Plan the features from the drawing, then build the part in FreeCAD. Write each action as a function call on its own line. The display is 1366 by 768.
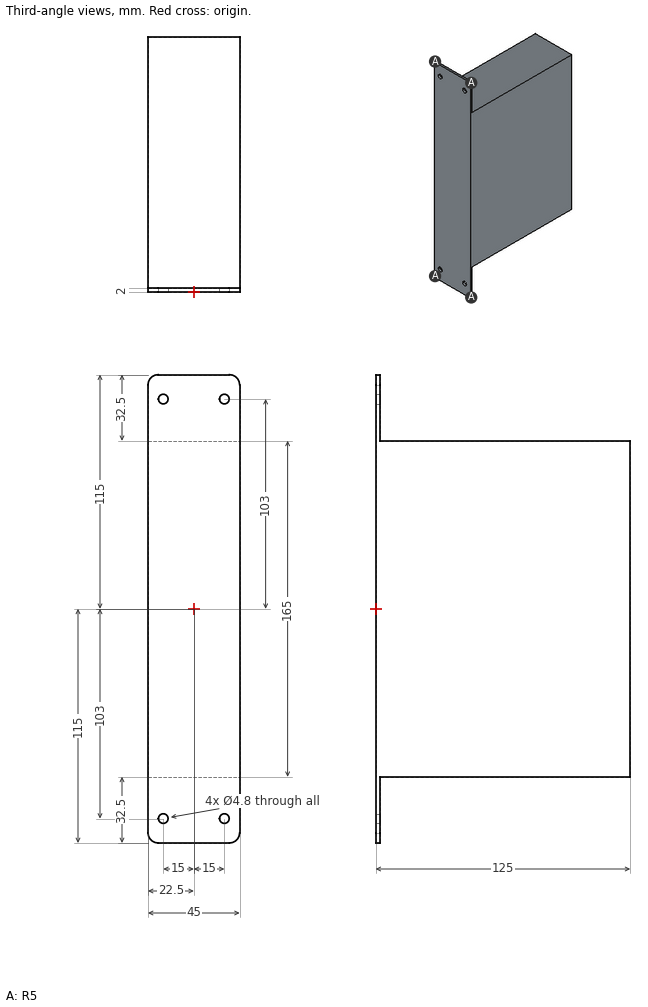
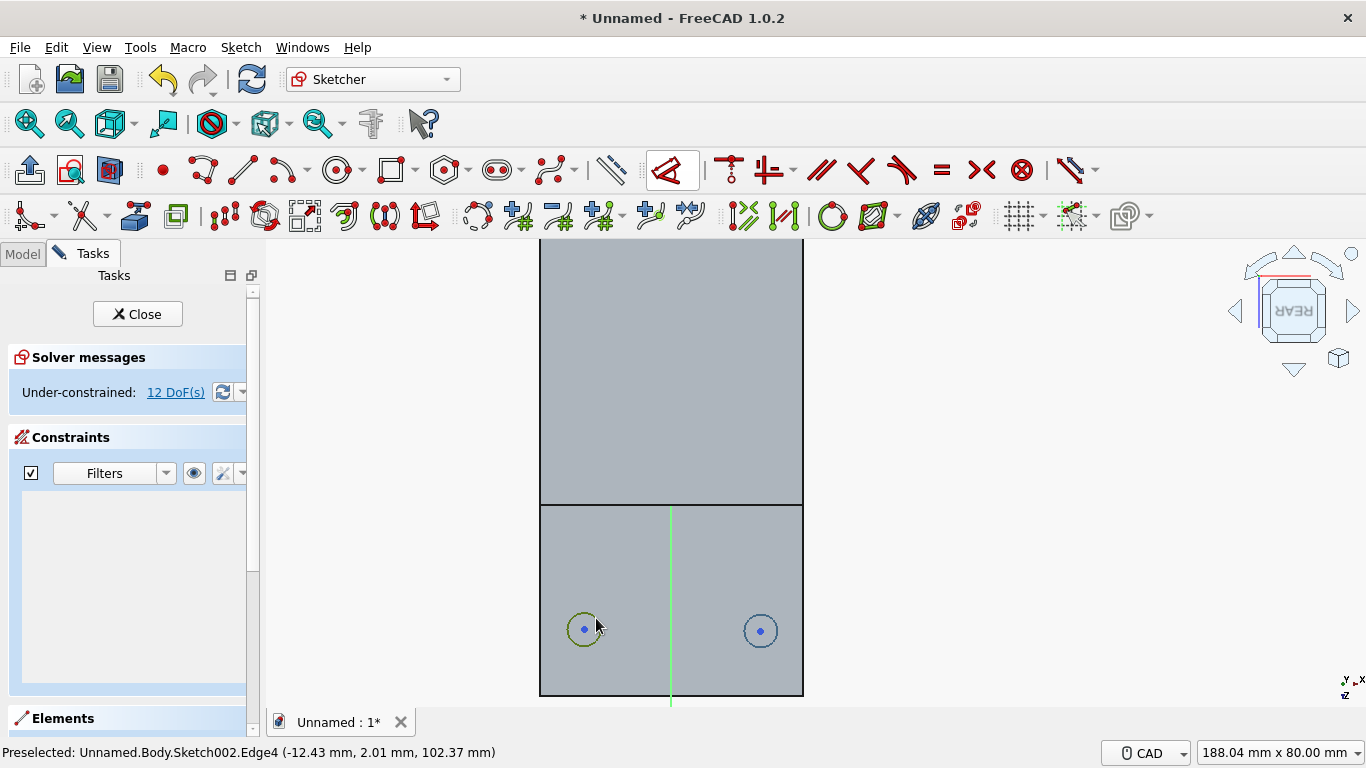
click(942, 170)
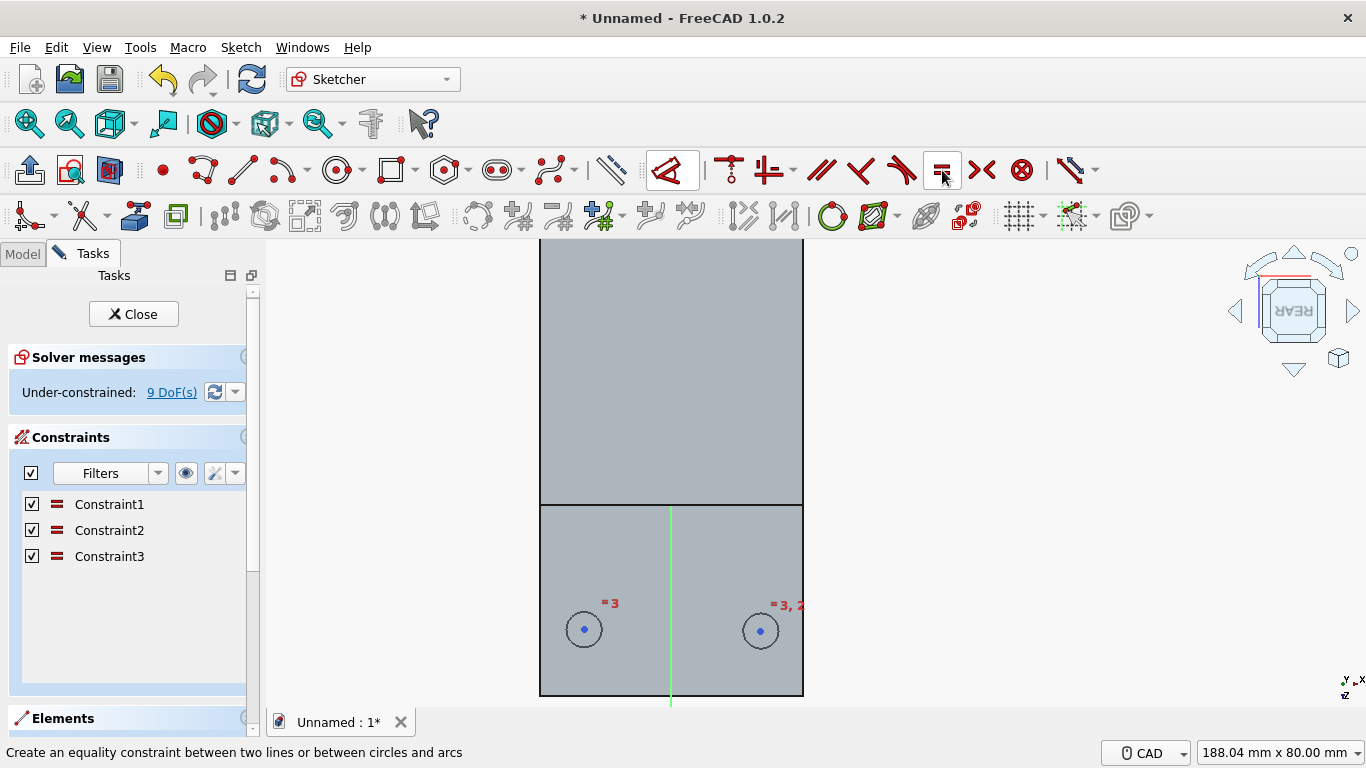
scroll(772, 620, down, 7)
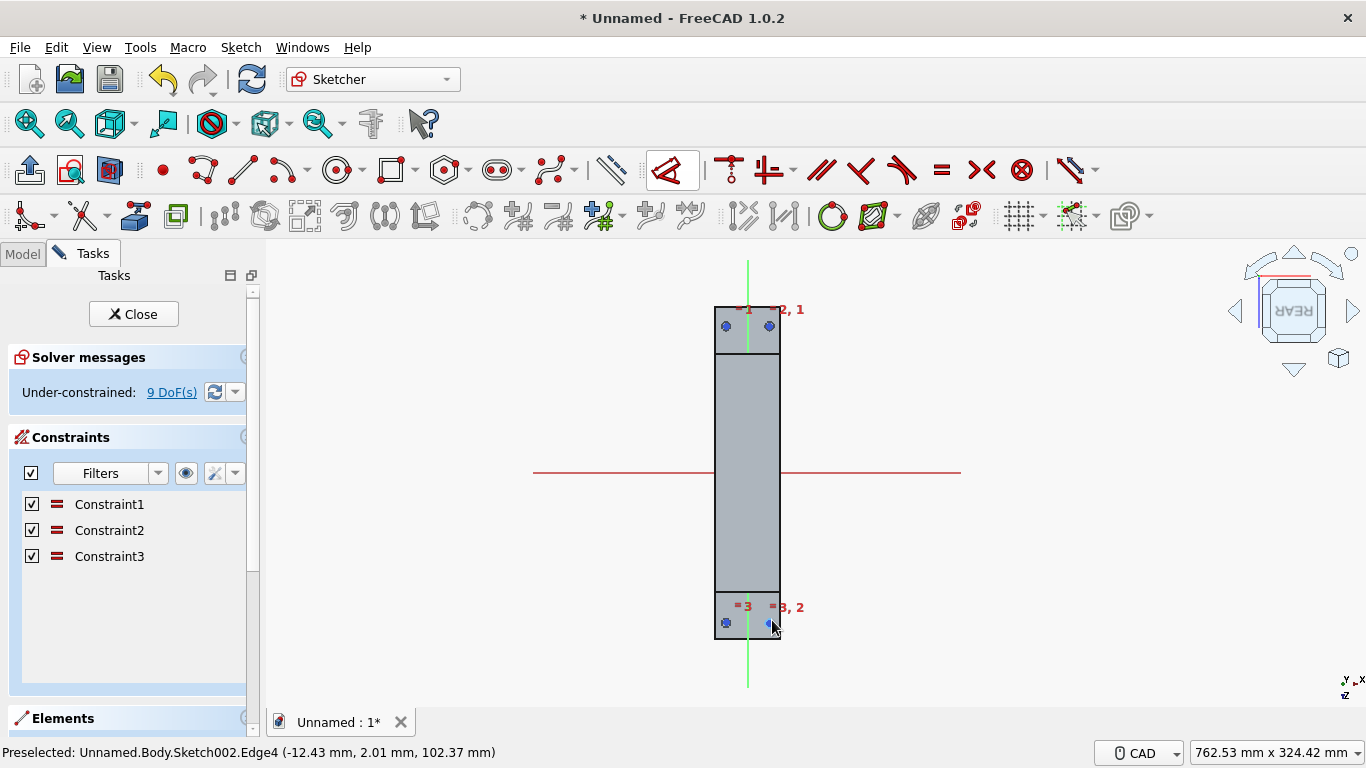
click(726, 326)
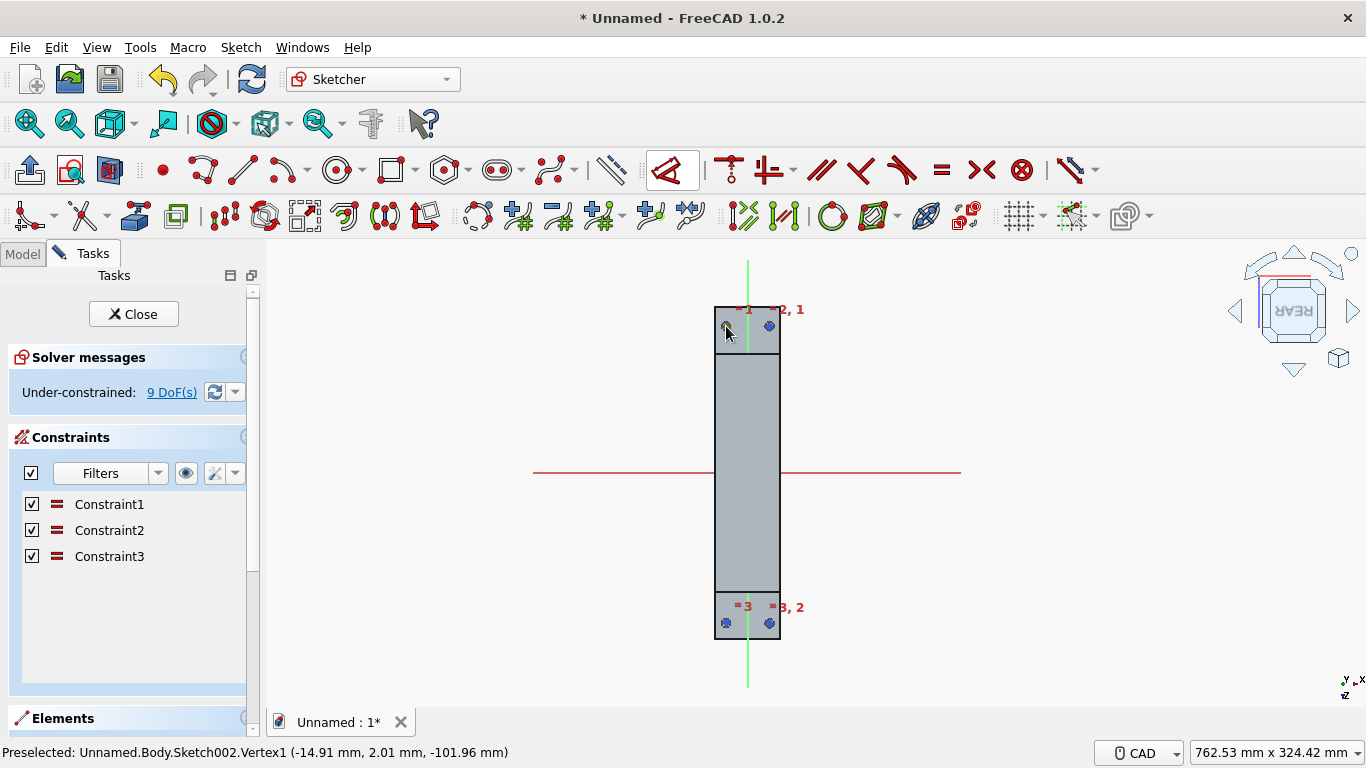
click(770, 326)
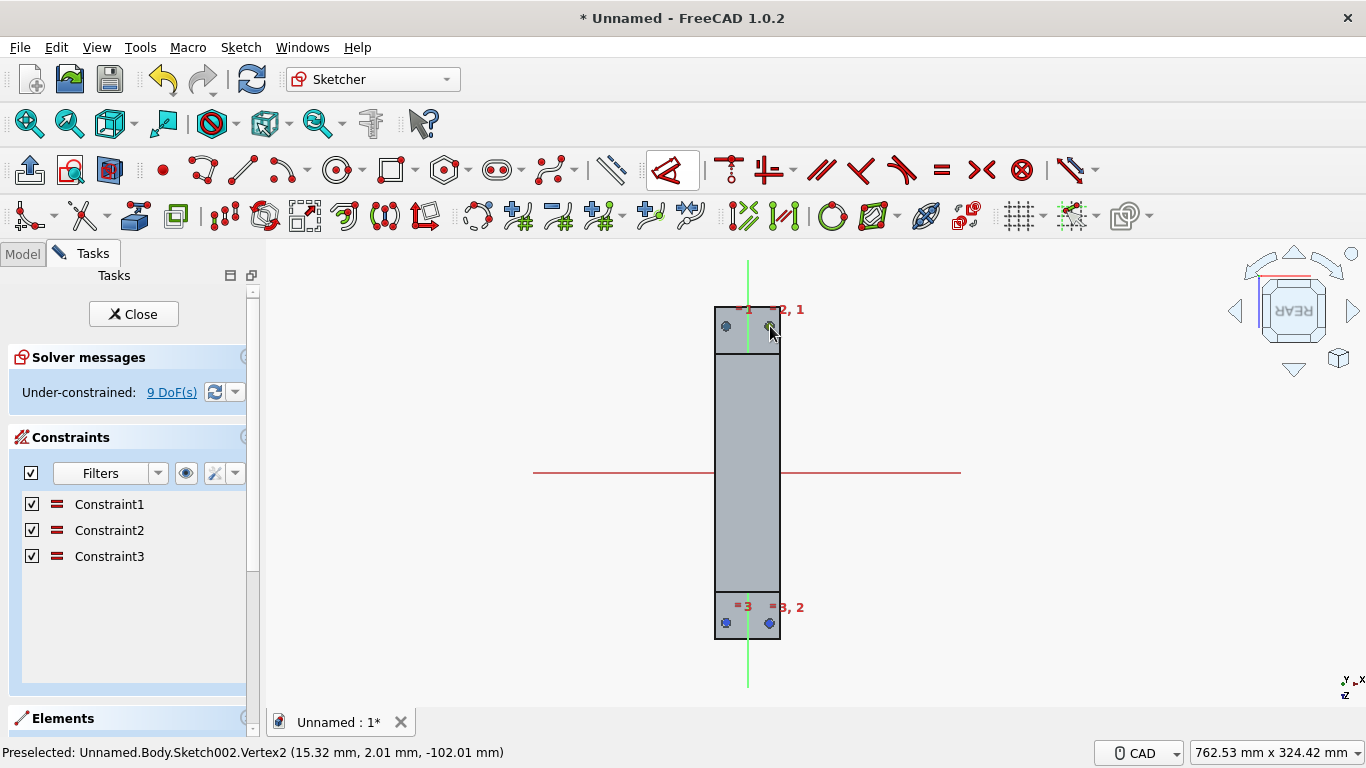
click(796, 170)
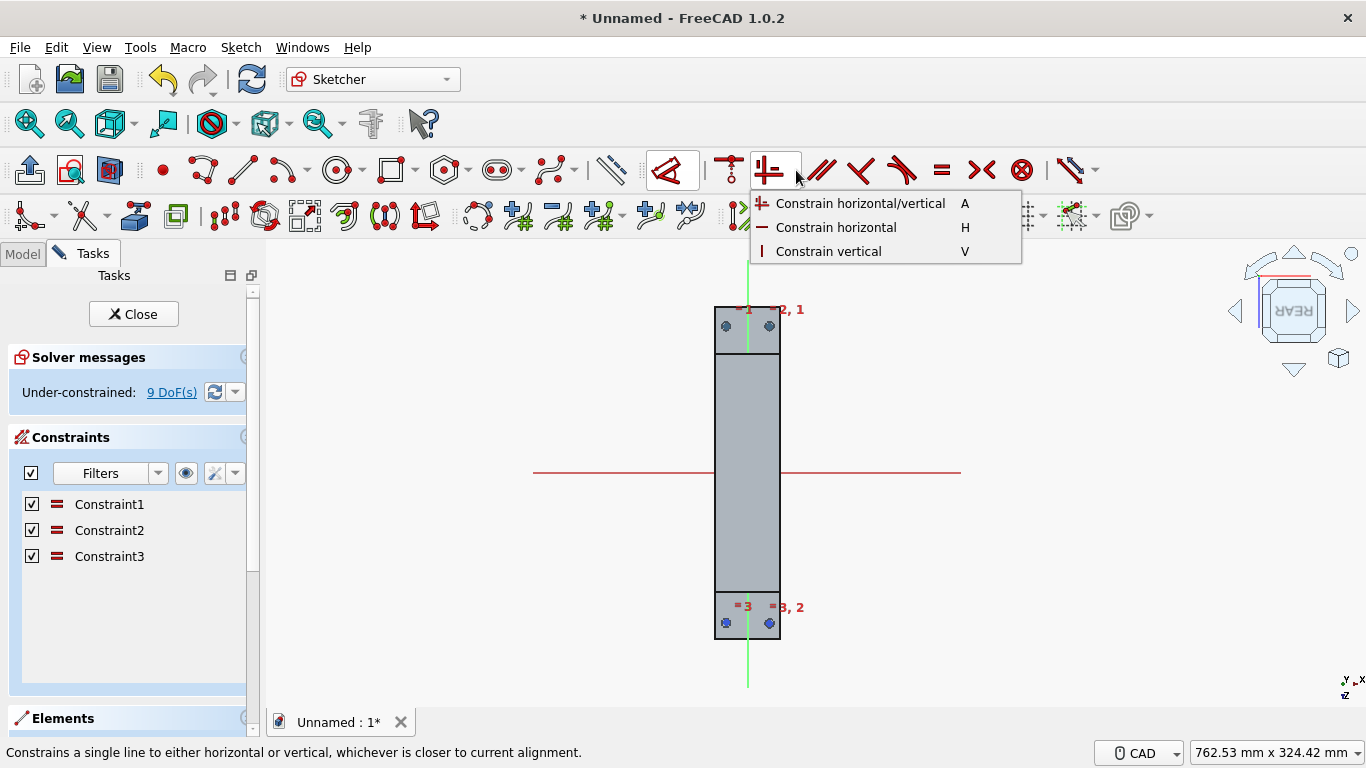
click(886, 227)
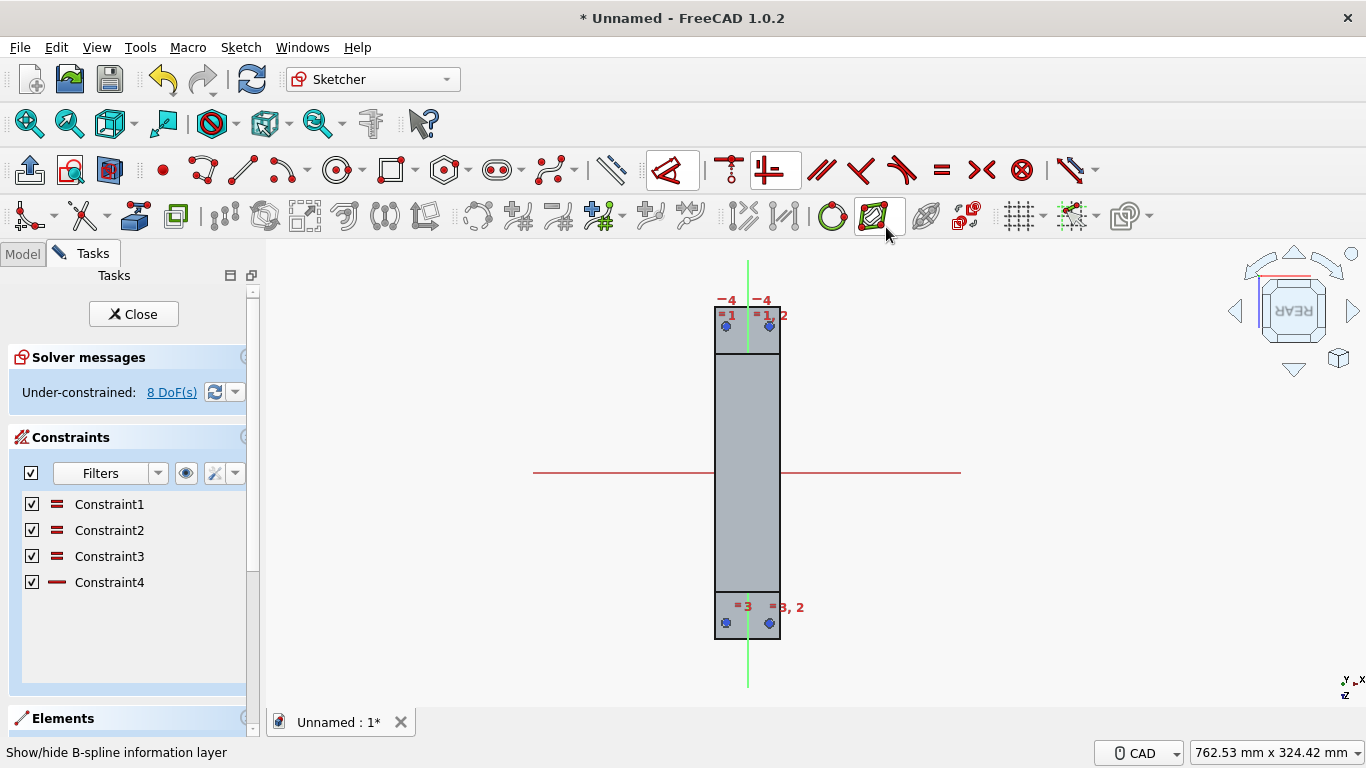
click(770, 326)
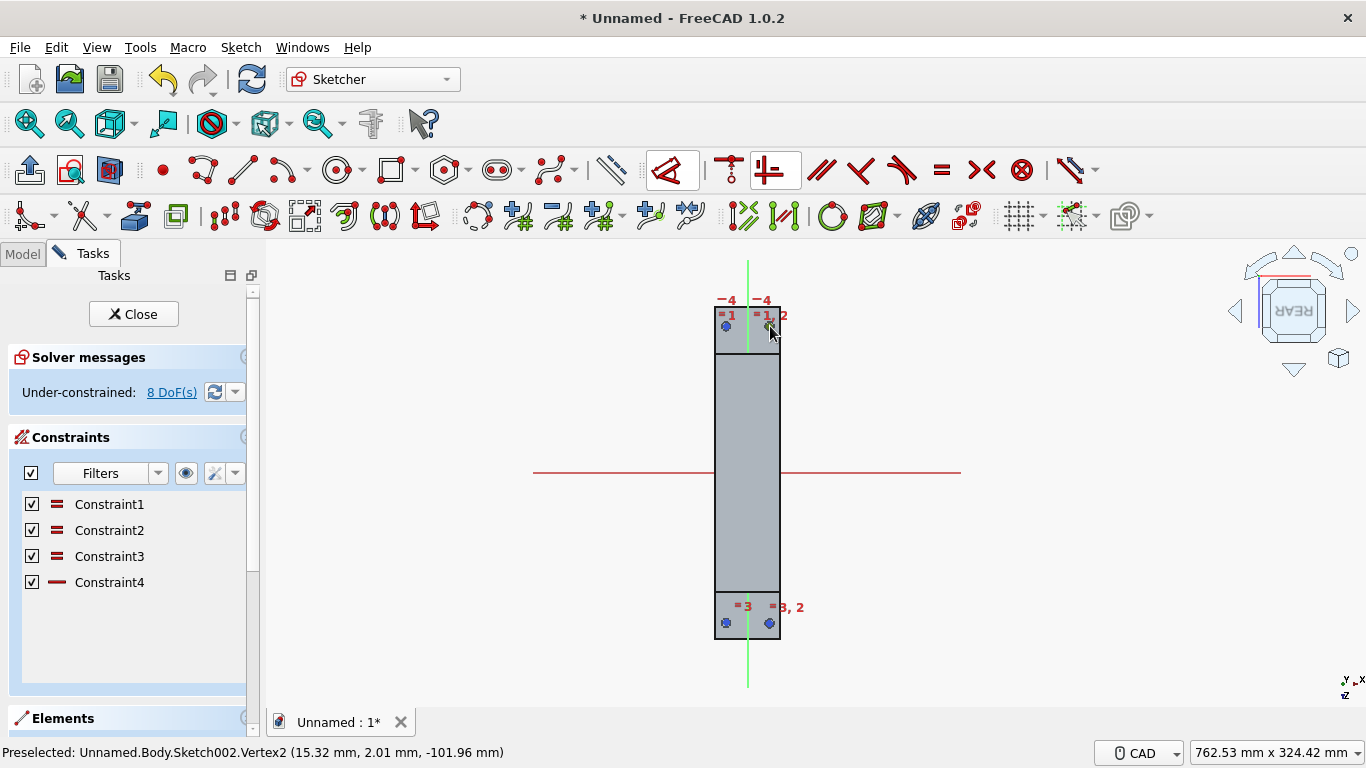
click(770, 623)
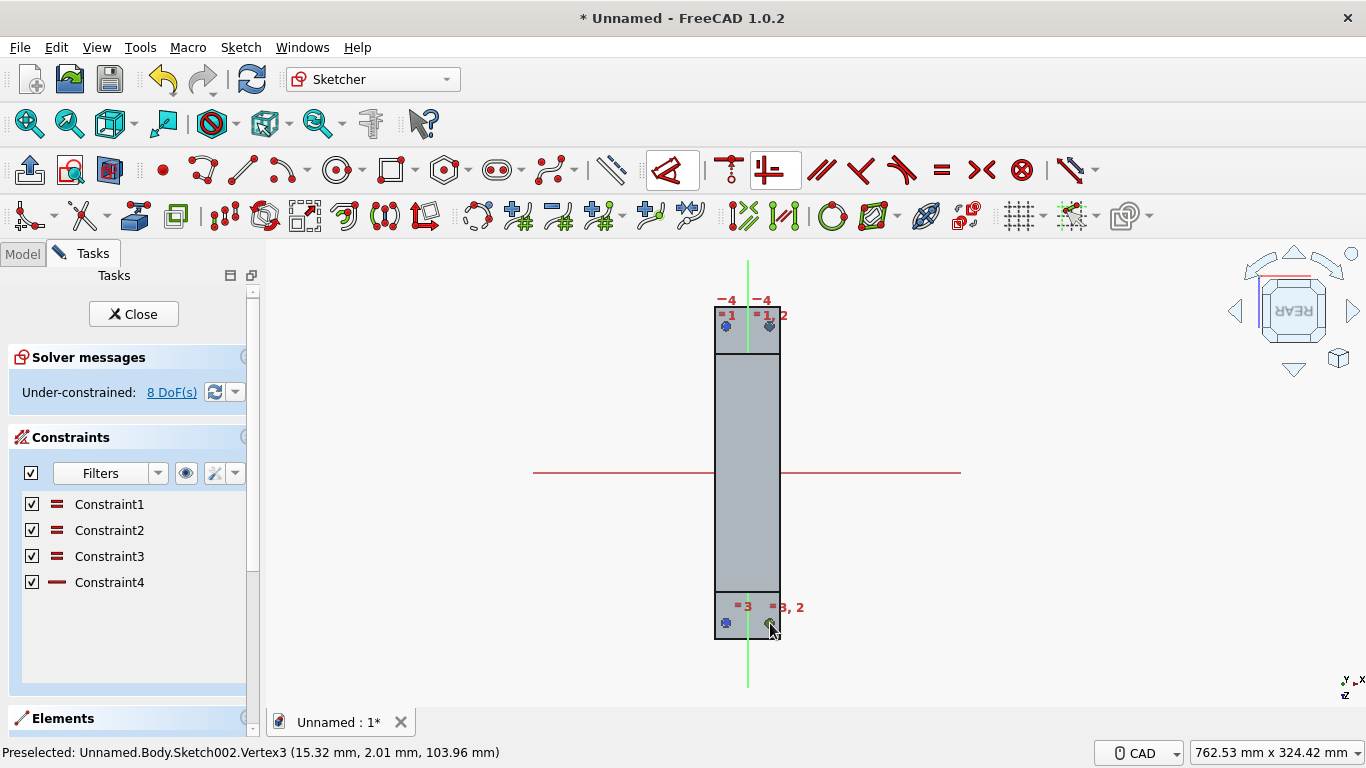
click(796, 170)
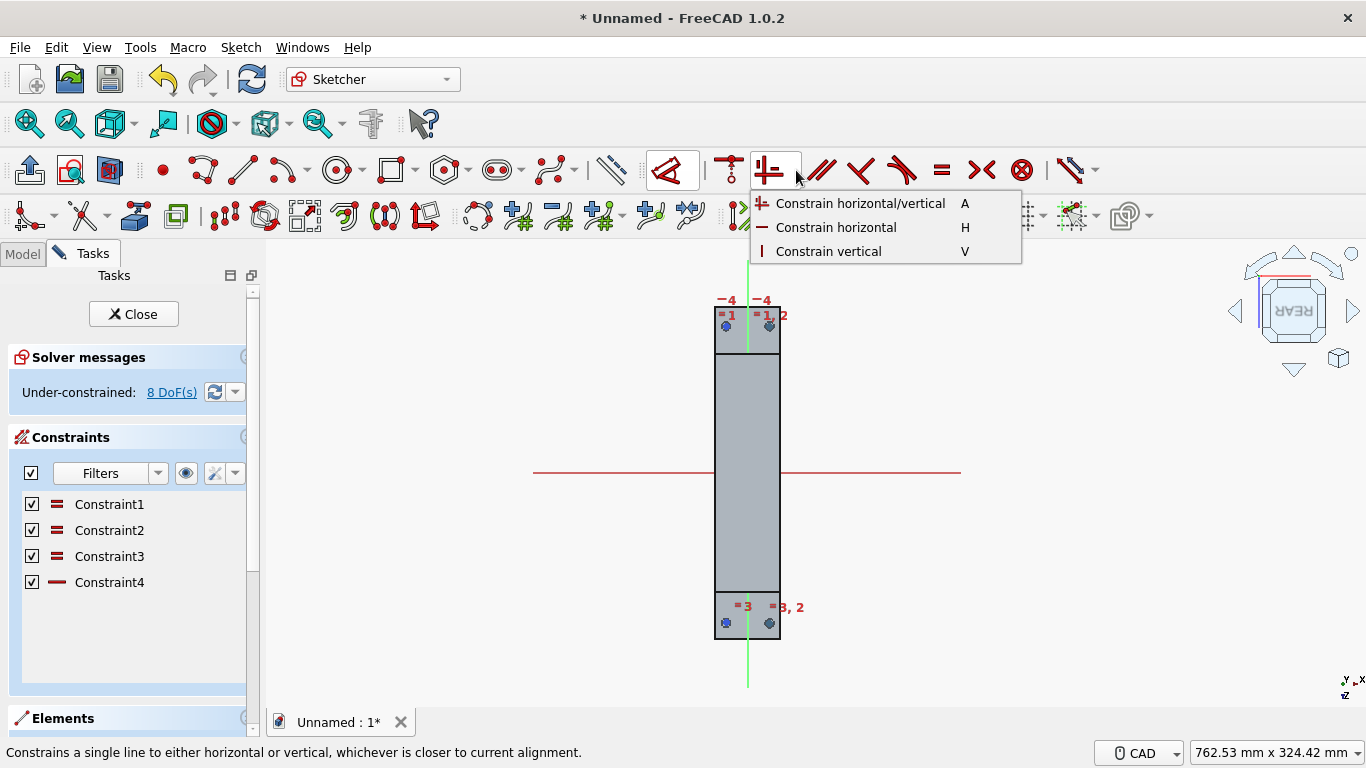
click(886, 251)